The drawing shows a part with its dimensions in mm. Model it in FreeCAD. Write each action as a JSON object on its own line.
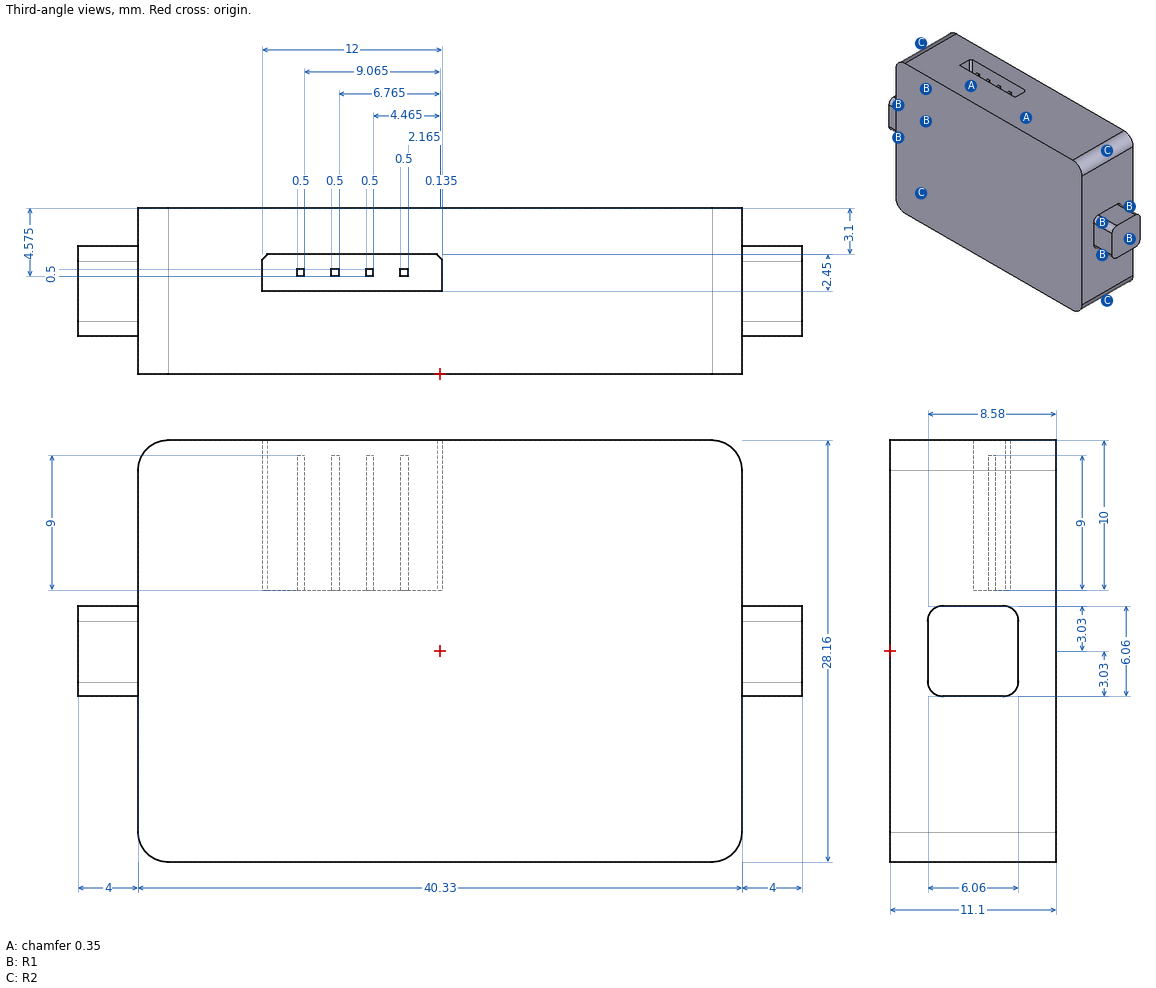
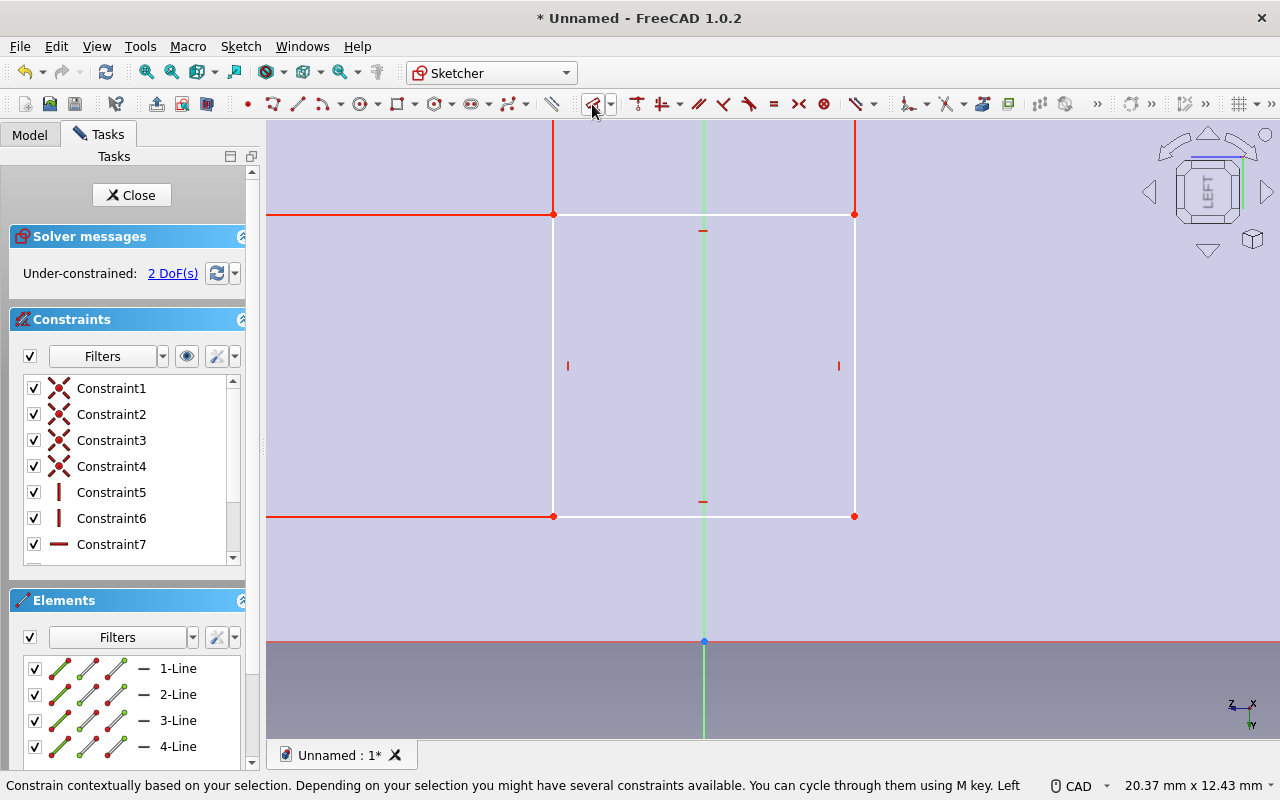
{"action": "left_click", "coordinate": [553, 215]}
{"action": "left_click", "coordinate": [629, 676]}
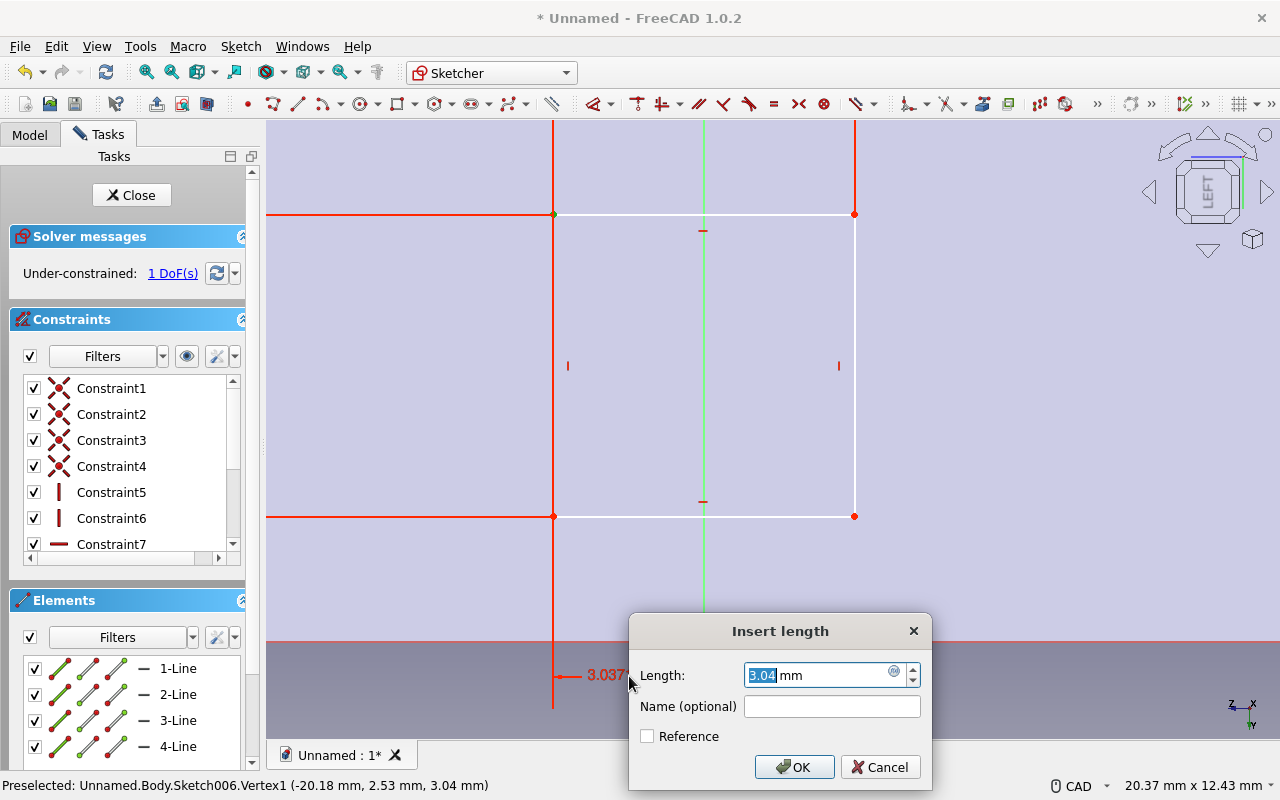
{"action": "type", "text": "3.03"}
{"action": "key", "text": "Return"}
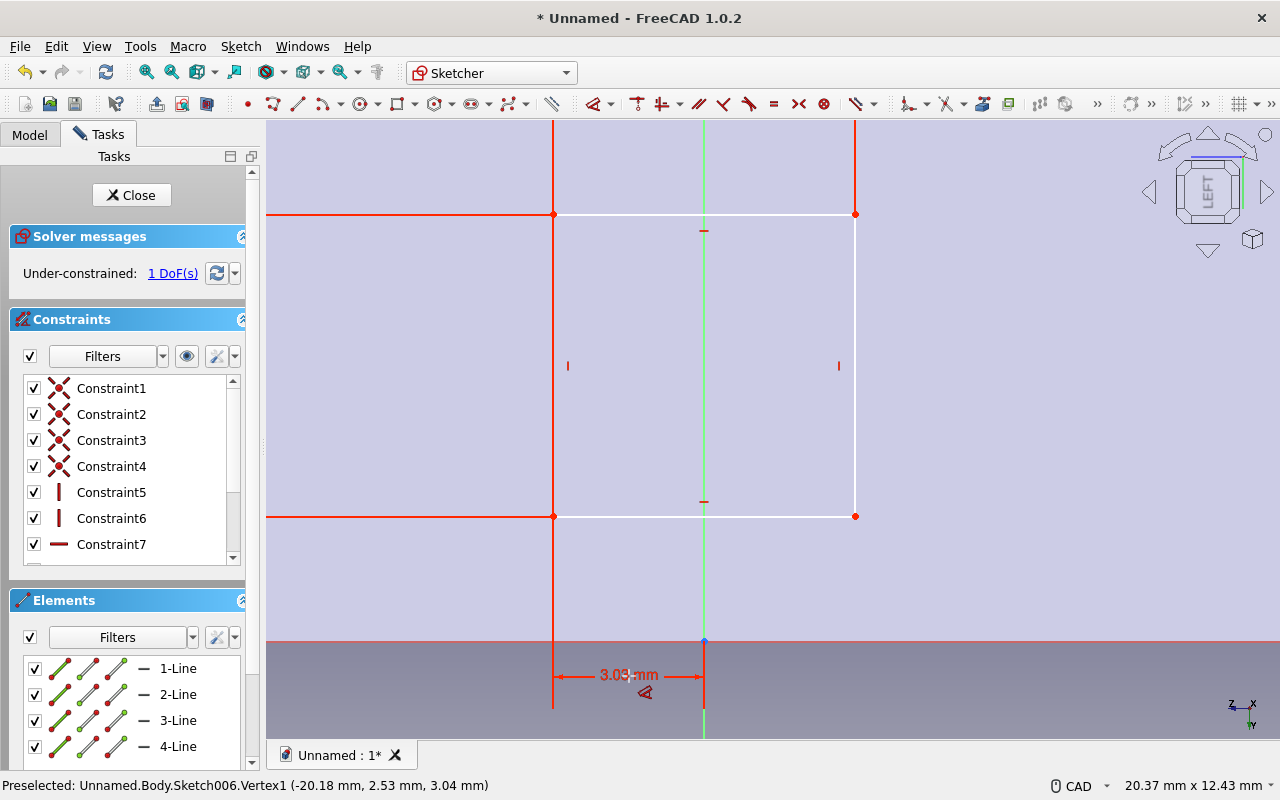
{"action": "left_click", "coordinate": [553, 215]}
{"action": "left_click", "coordinate": [519, 428]}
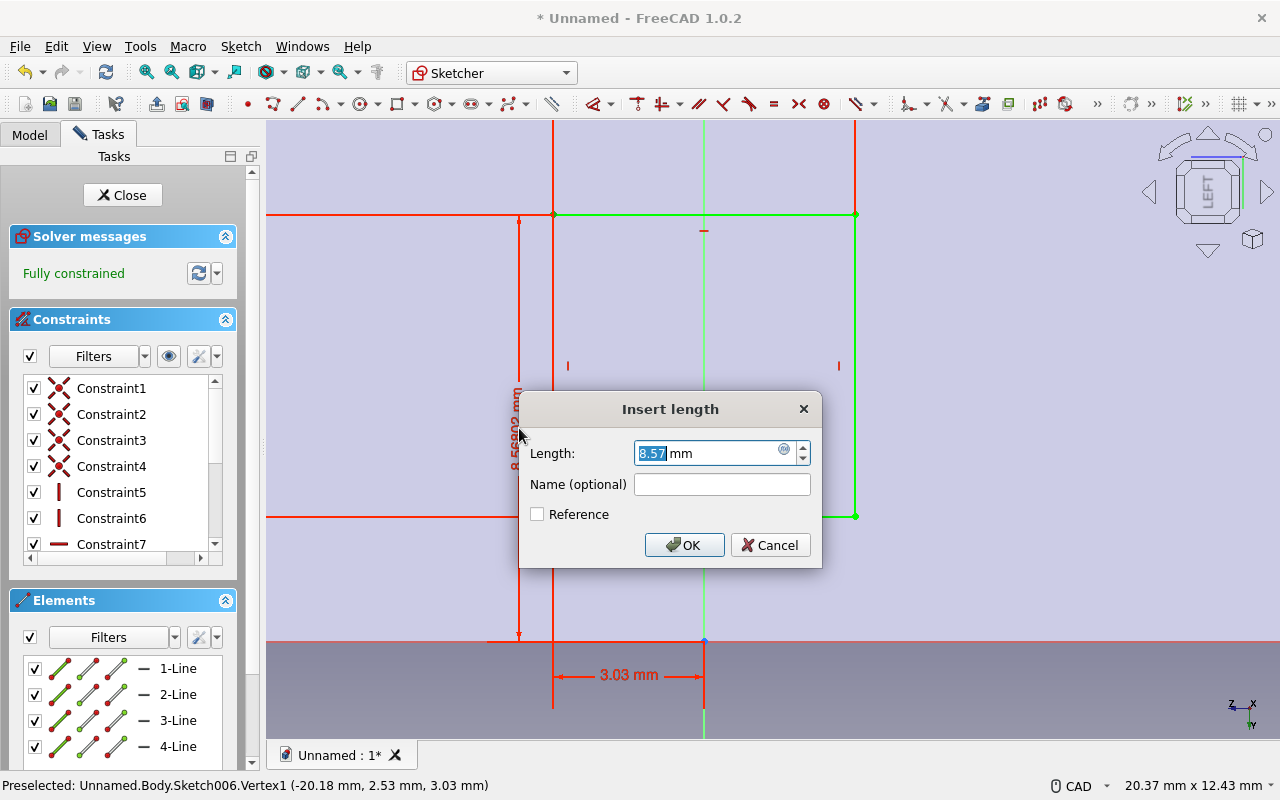
{"action": "type", "text": "8.58"}
{"action": "key", "text": "Return"}
{"action": "key", "text": "Escape"}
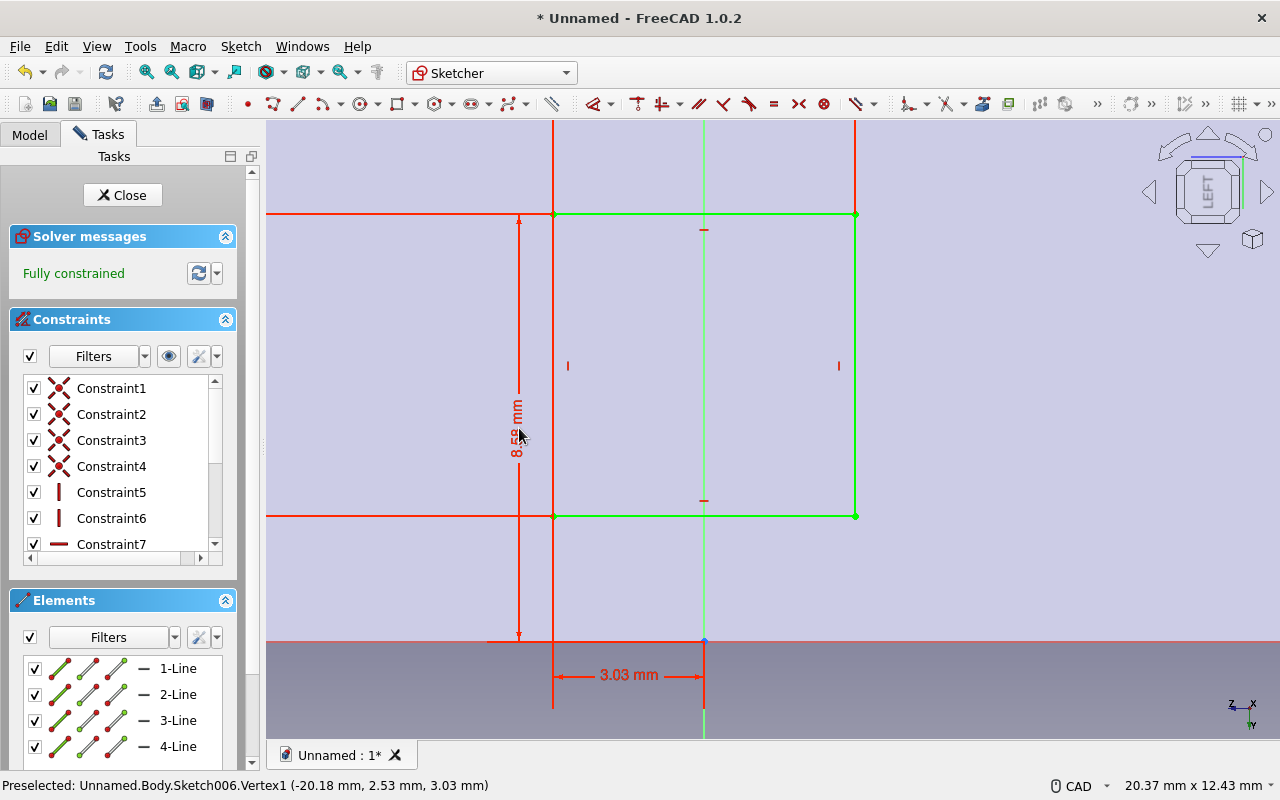
{"action": "left_click", "coordinate": [123, 195]}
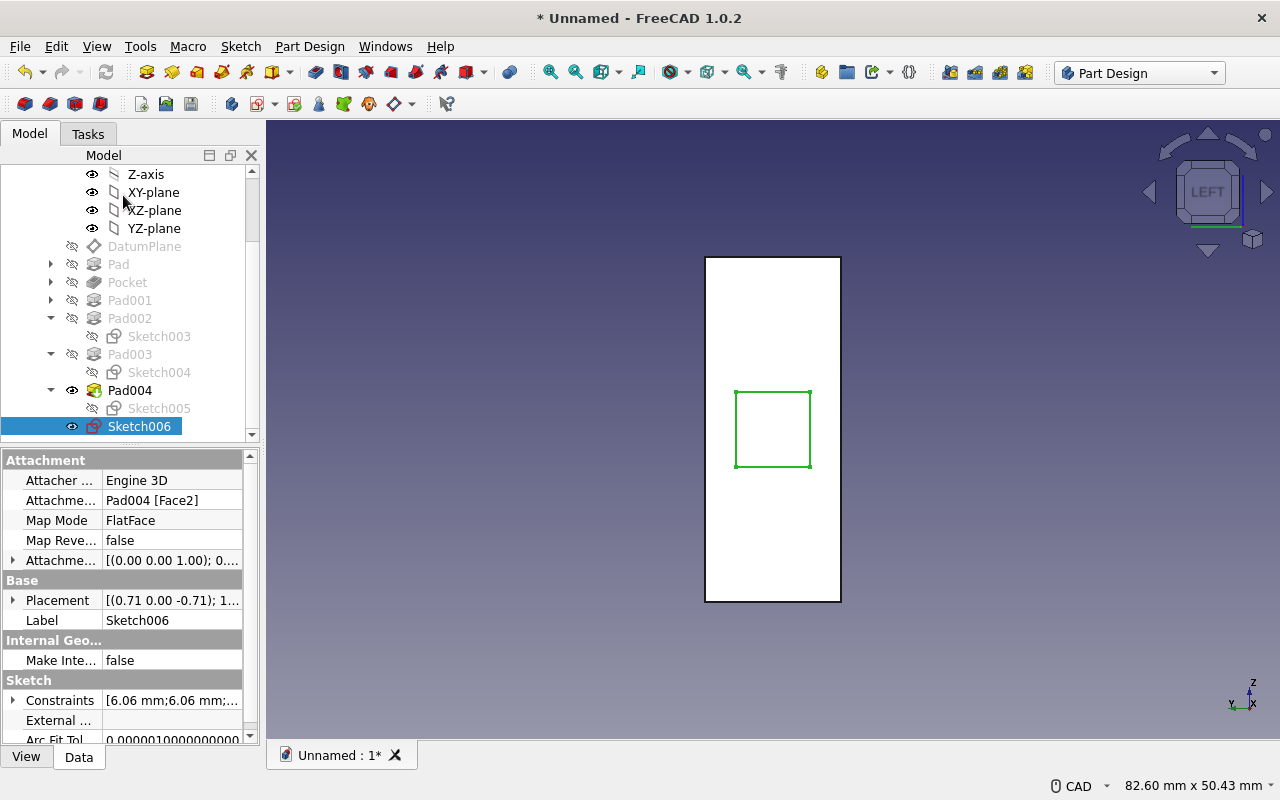
{"action": "left_click", "coordinate": [147, 72]}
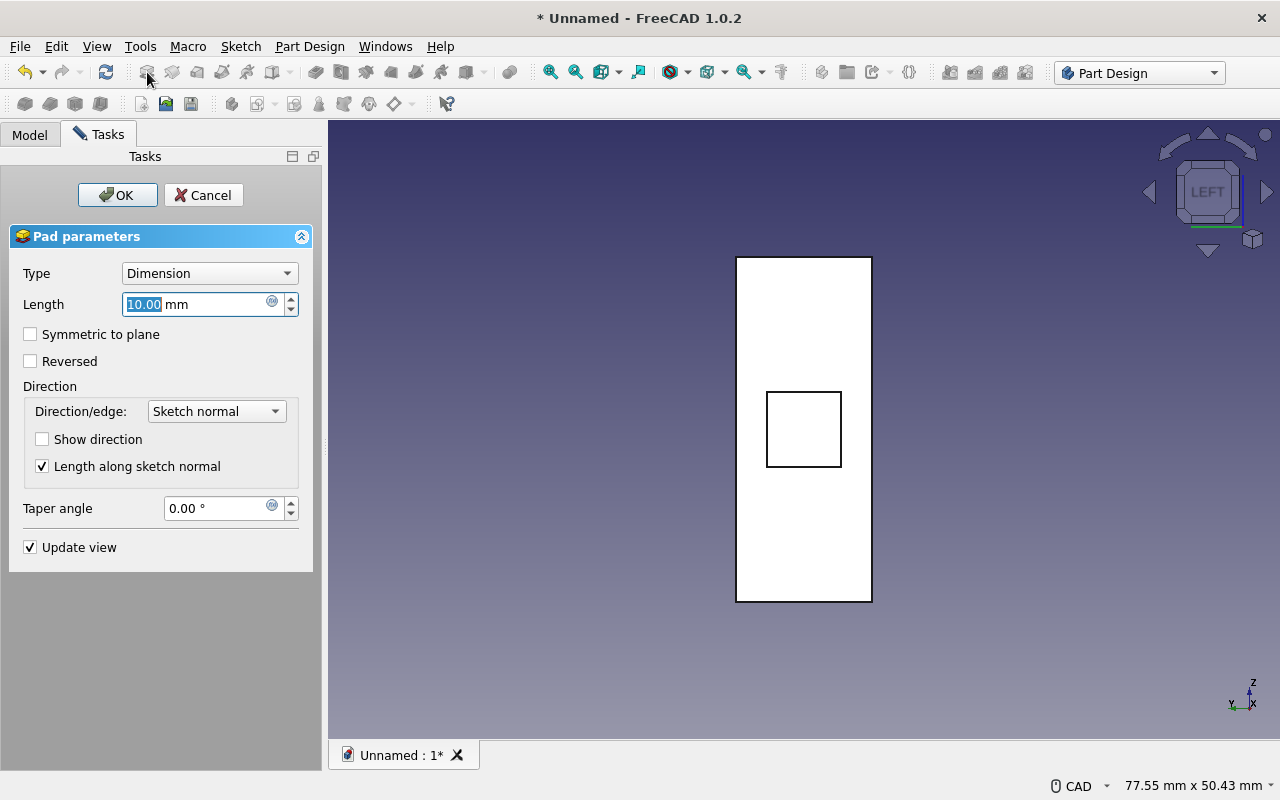
{"action": "type", "text": "4"}
{"action": "key", "text": "Tab"}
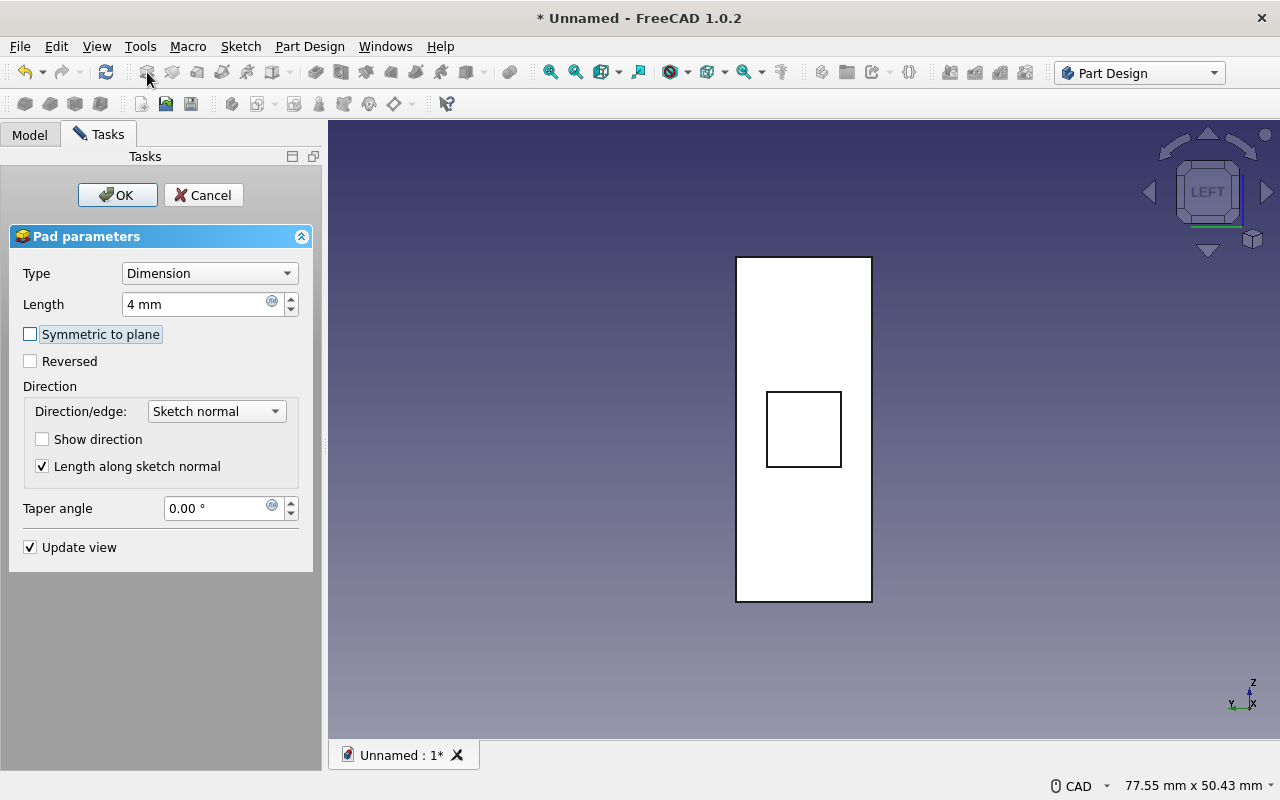
{"action": "left_click", "coordinate": [118, 195]}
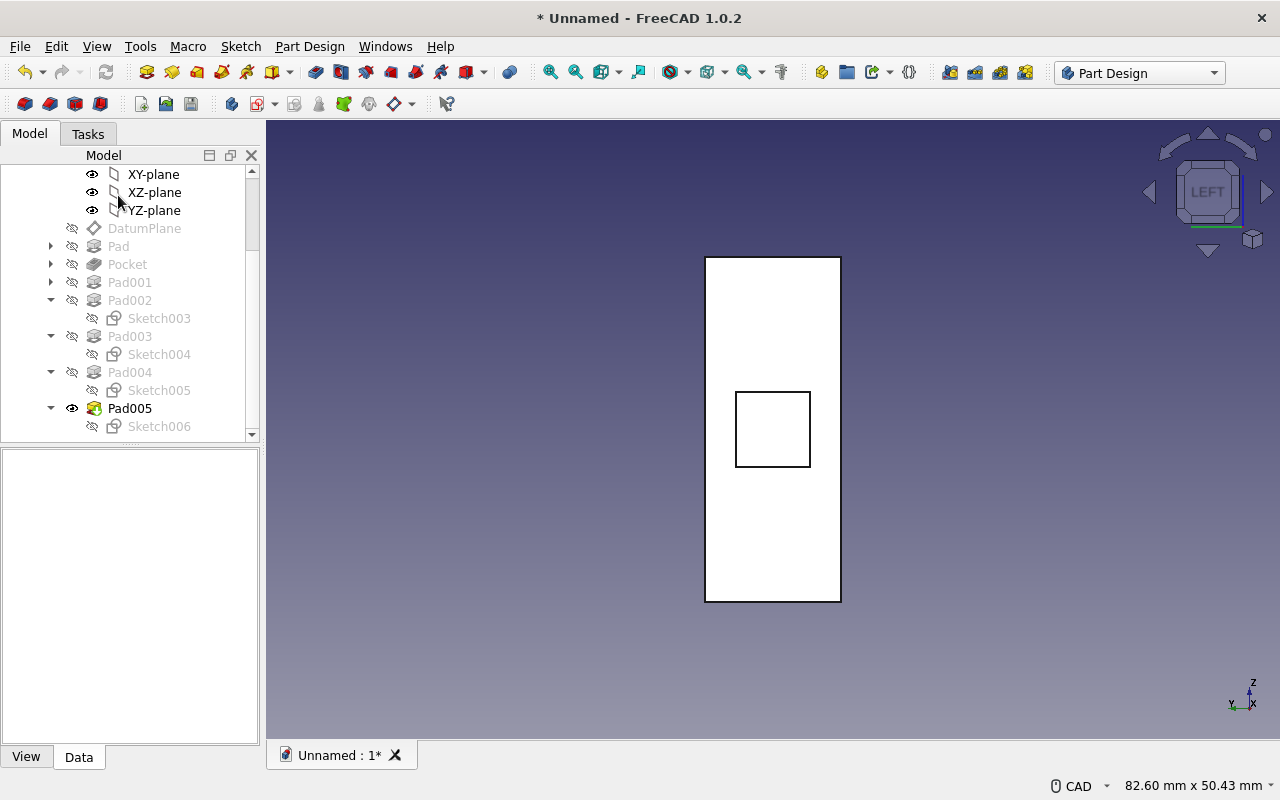
{"action": "key", "text": "0"}